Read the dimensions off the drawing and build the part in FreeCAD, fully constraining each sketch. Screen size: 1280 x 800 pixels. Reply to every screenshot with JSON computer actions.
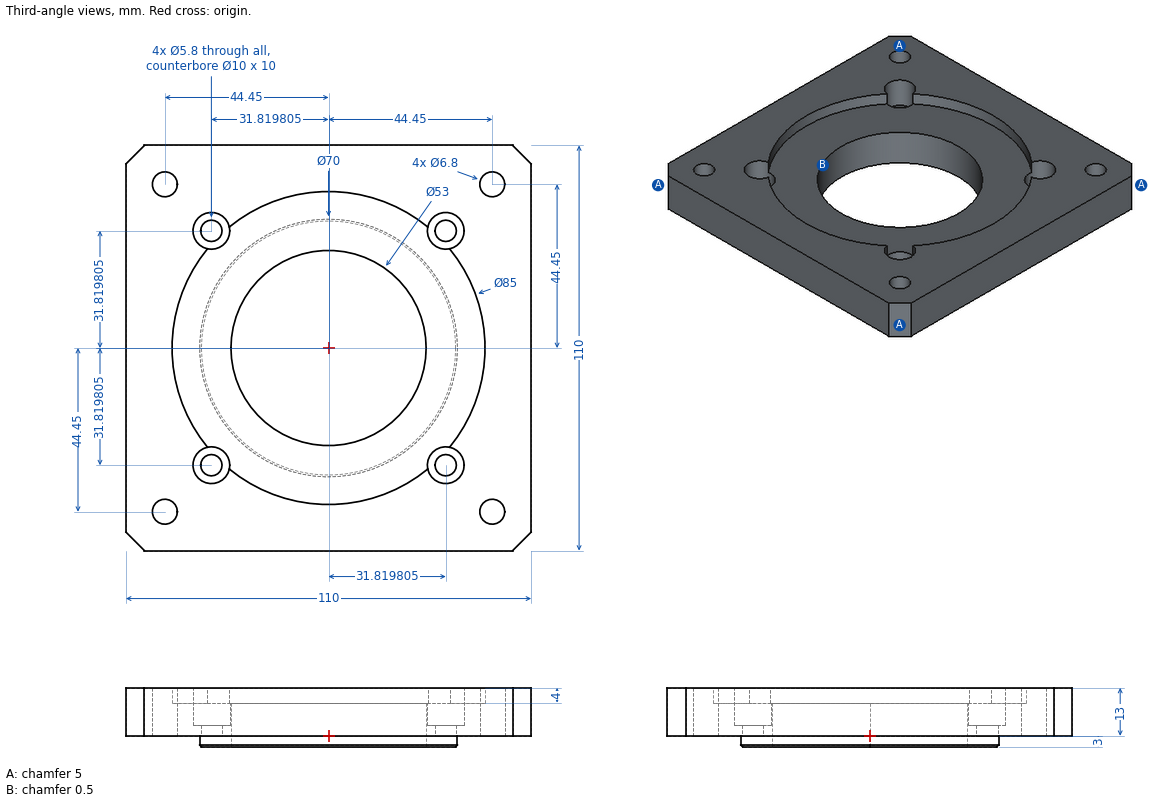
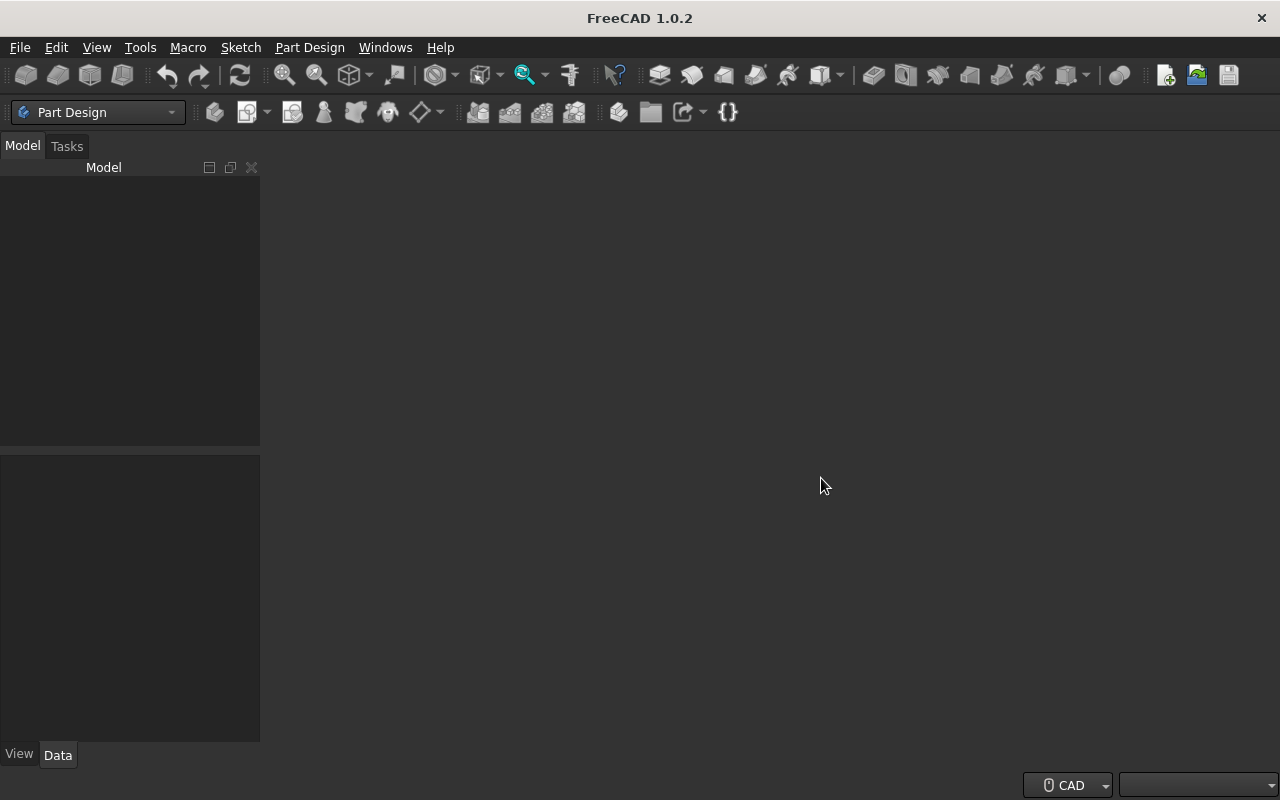
{"action": "left_click", "coordinate": [1166, 76]}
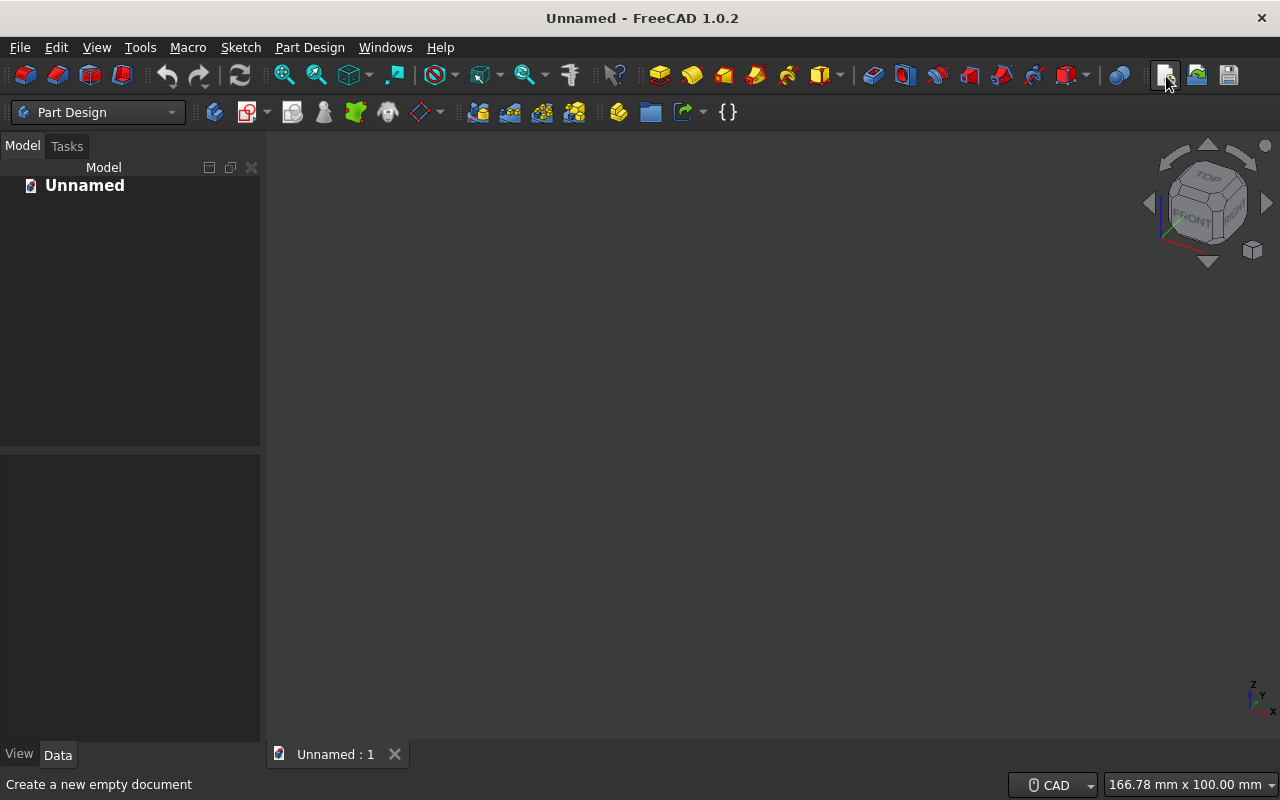
{"action": "left_click", "coordinate": [248, 112]}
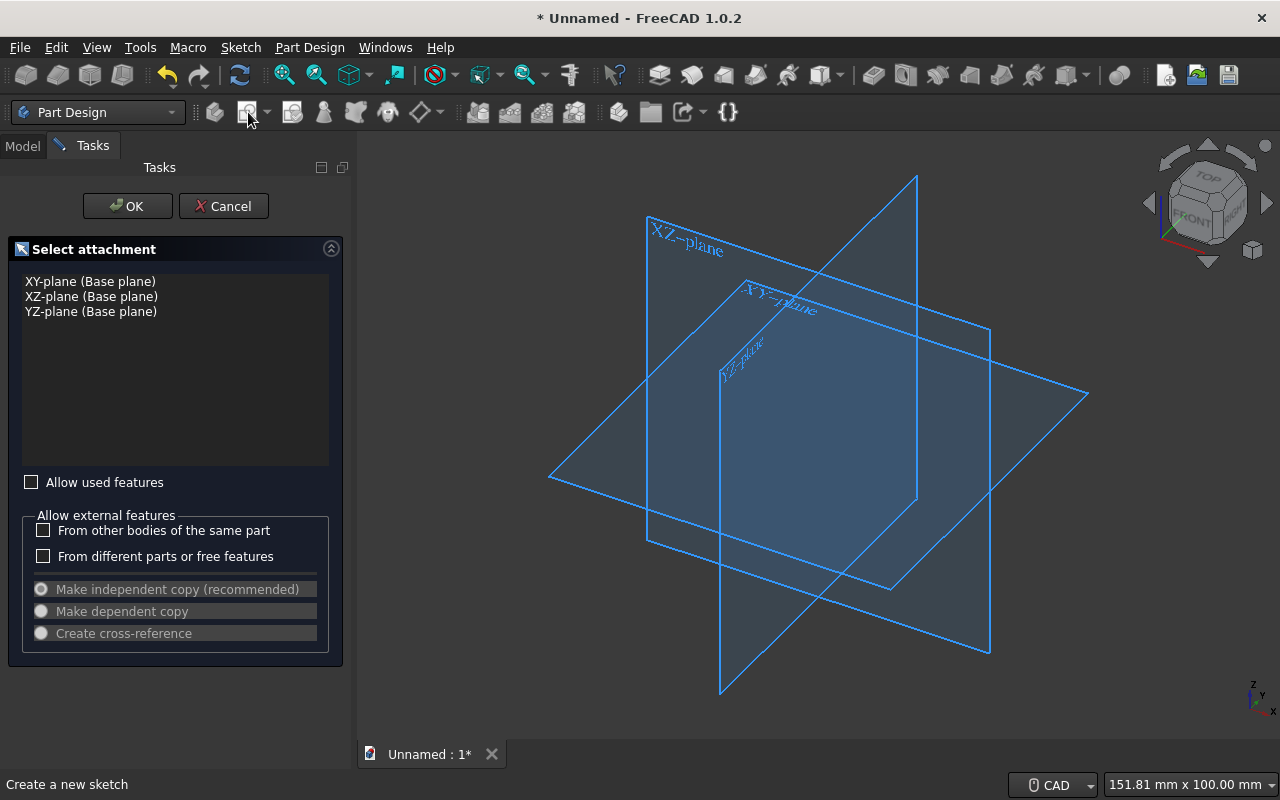
{"action": "left_click", "coordinate": [82, 282]}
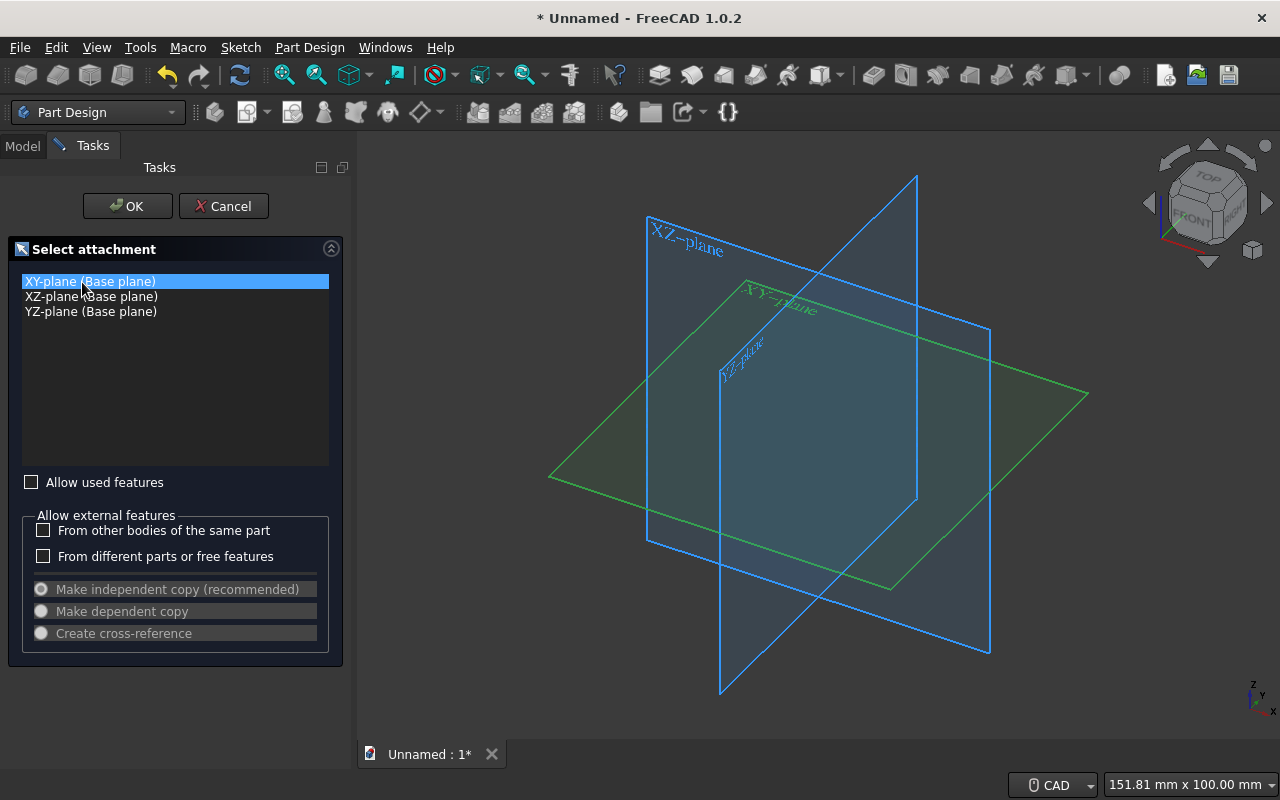
{"action": "left_click", "coordinate": [128, 206]}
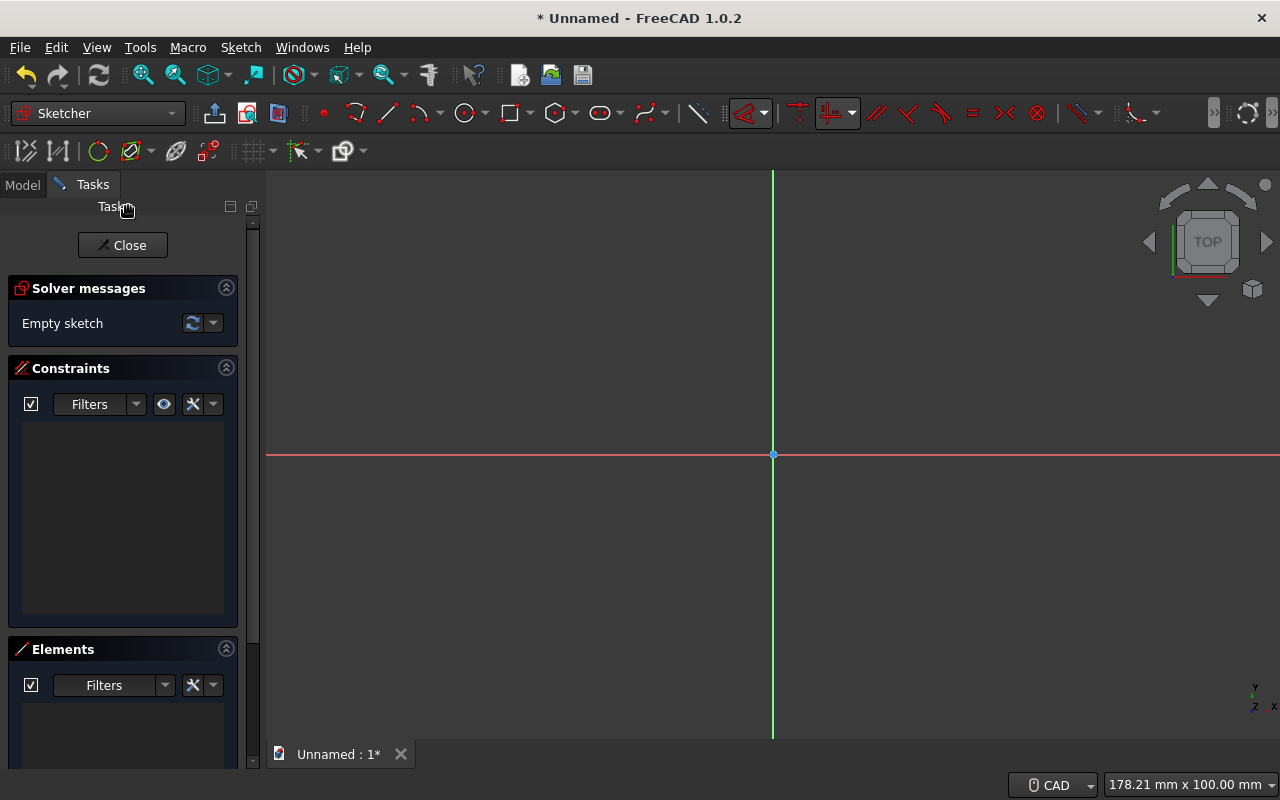
{"action": "scroll", "coordinate": [621, 454], "scroll_direction": "down", "scroll_amount": 3}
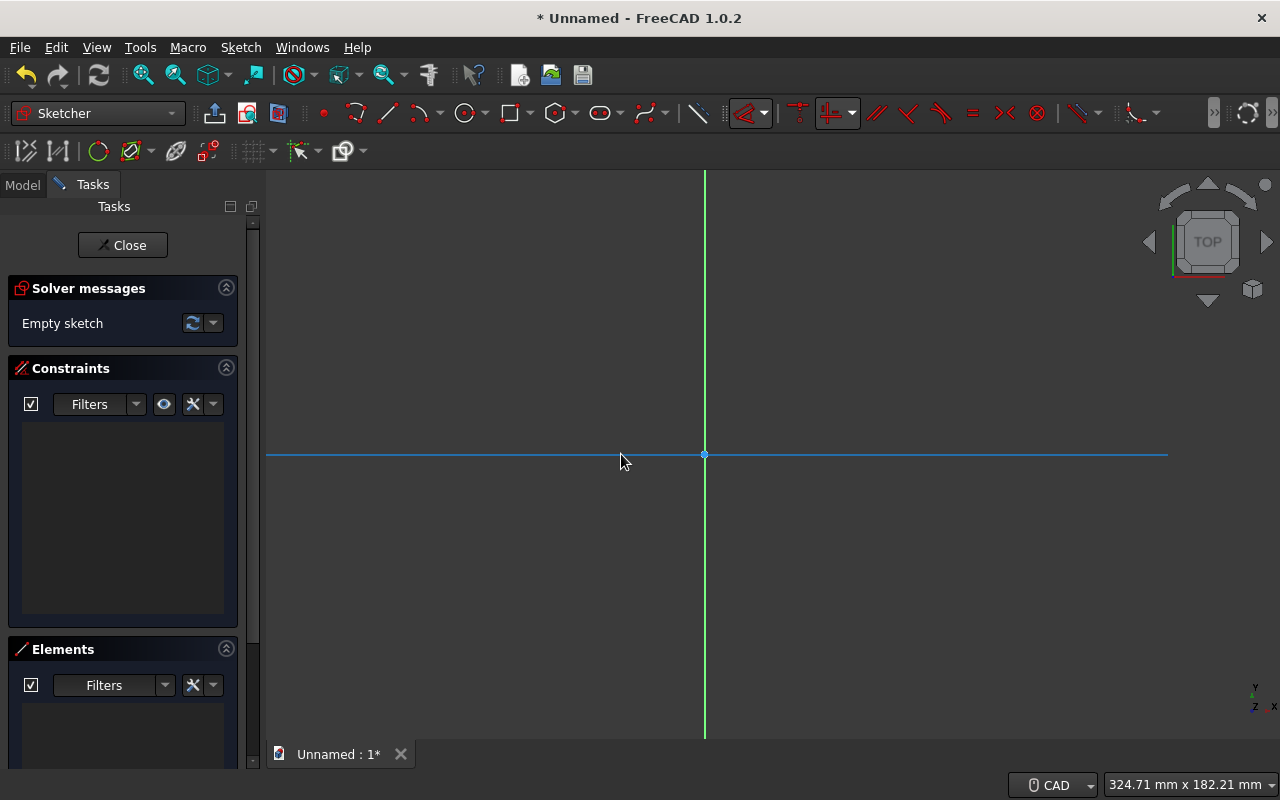
{"action": "key", "text": "g v"}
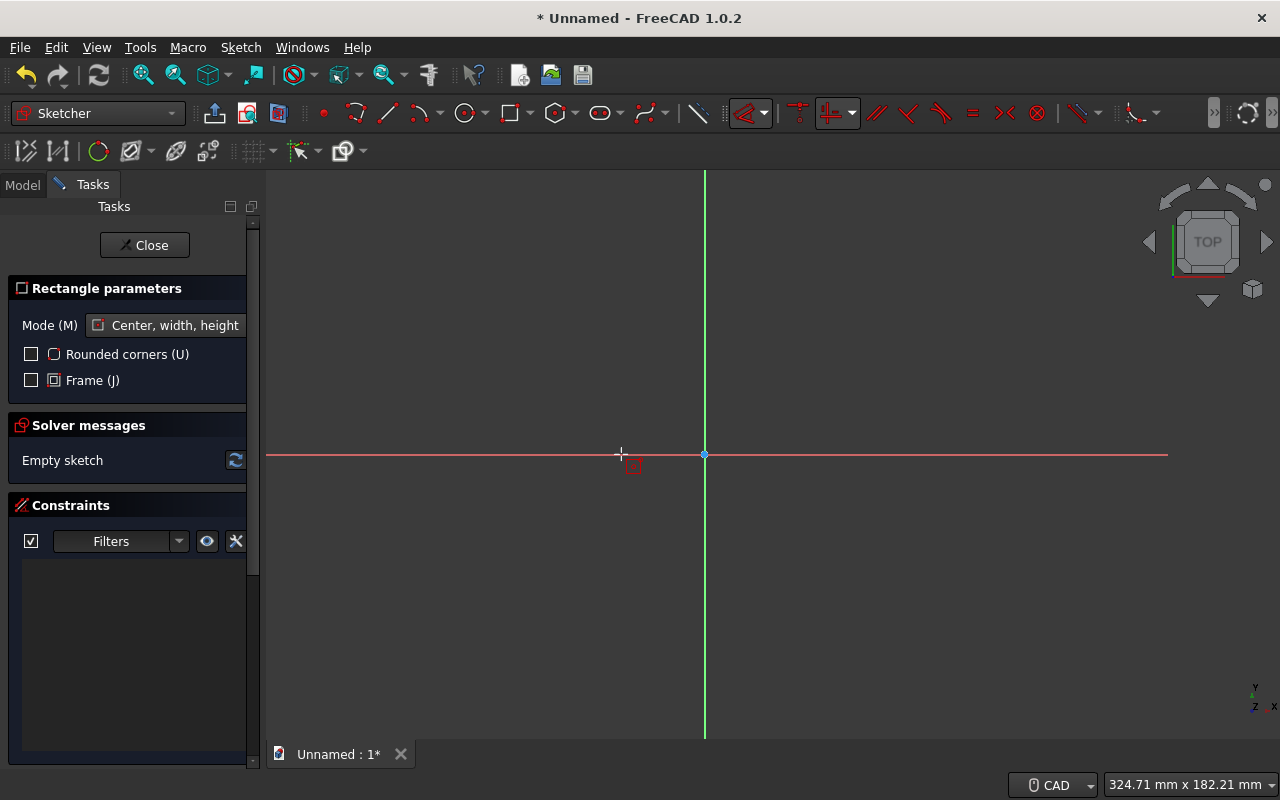
{"action": "left_click", "coordinate": [705, 454]}
{"action": "left_click", "coordinate": [876, 283]}
{"action": "key", "text": "Escape"}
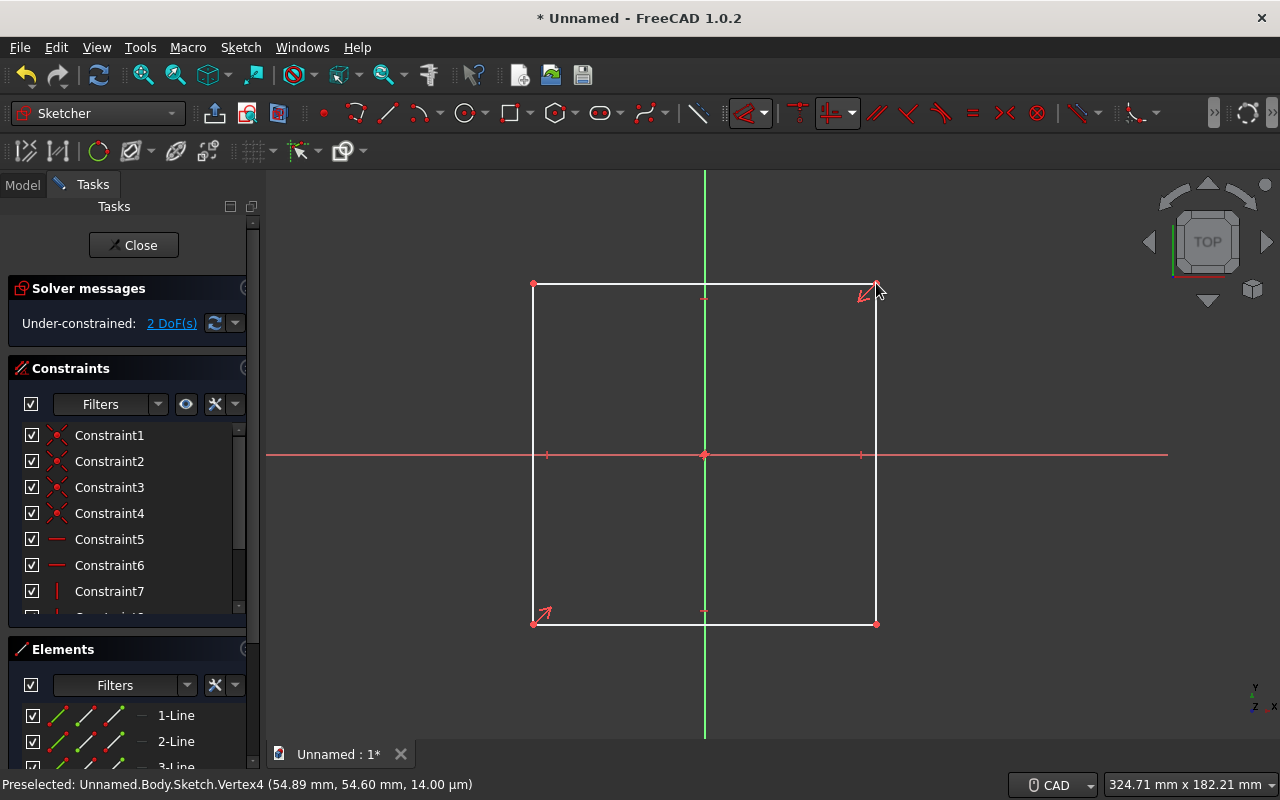
{"action": "left_click", "coordinate": [636, 625]}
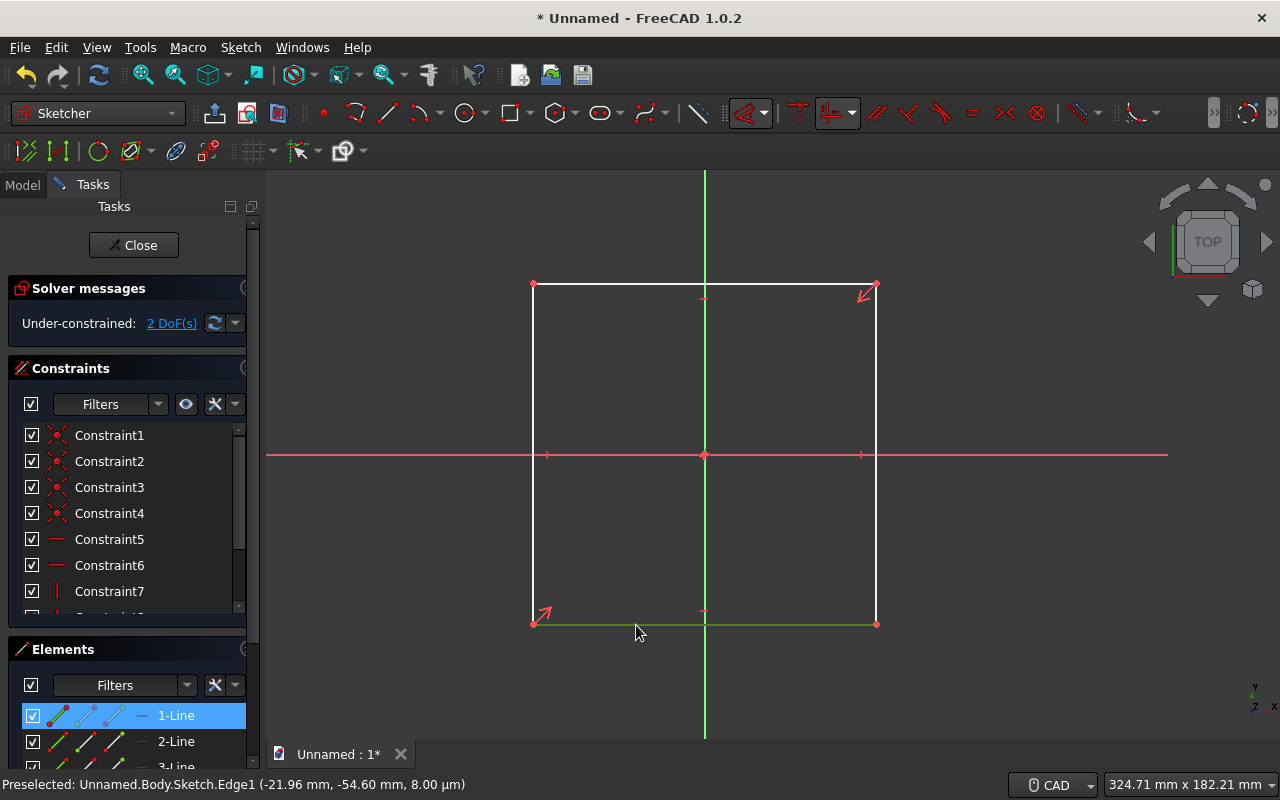
{"action": "left_click", "coordinate": [766, 114]}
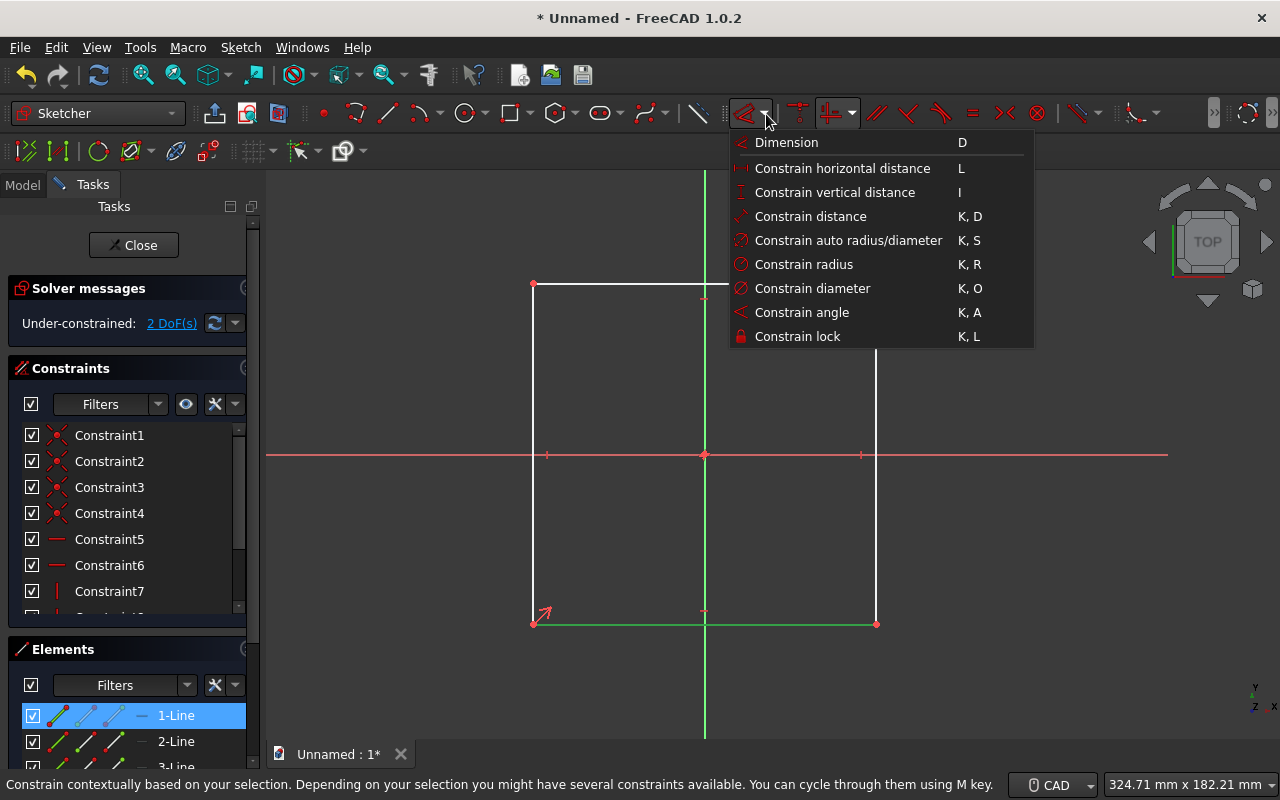
{"action": "left_click", "coordinate": [882, 168]}